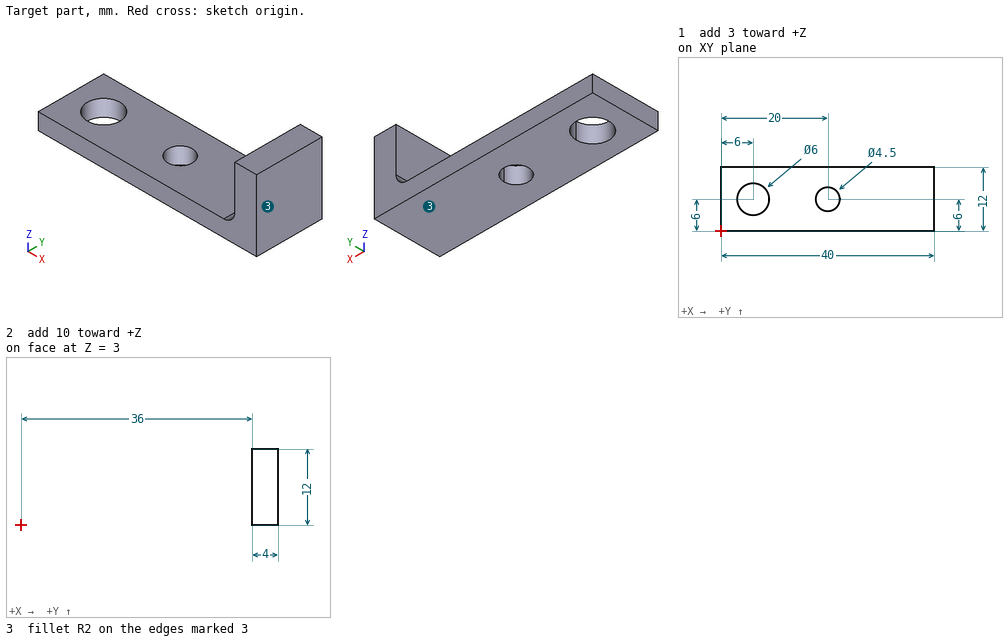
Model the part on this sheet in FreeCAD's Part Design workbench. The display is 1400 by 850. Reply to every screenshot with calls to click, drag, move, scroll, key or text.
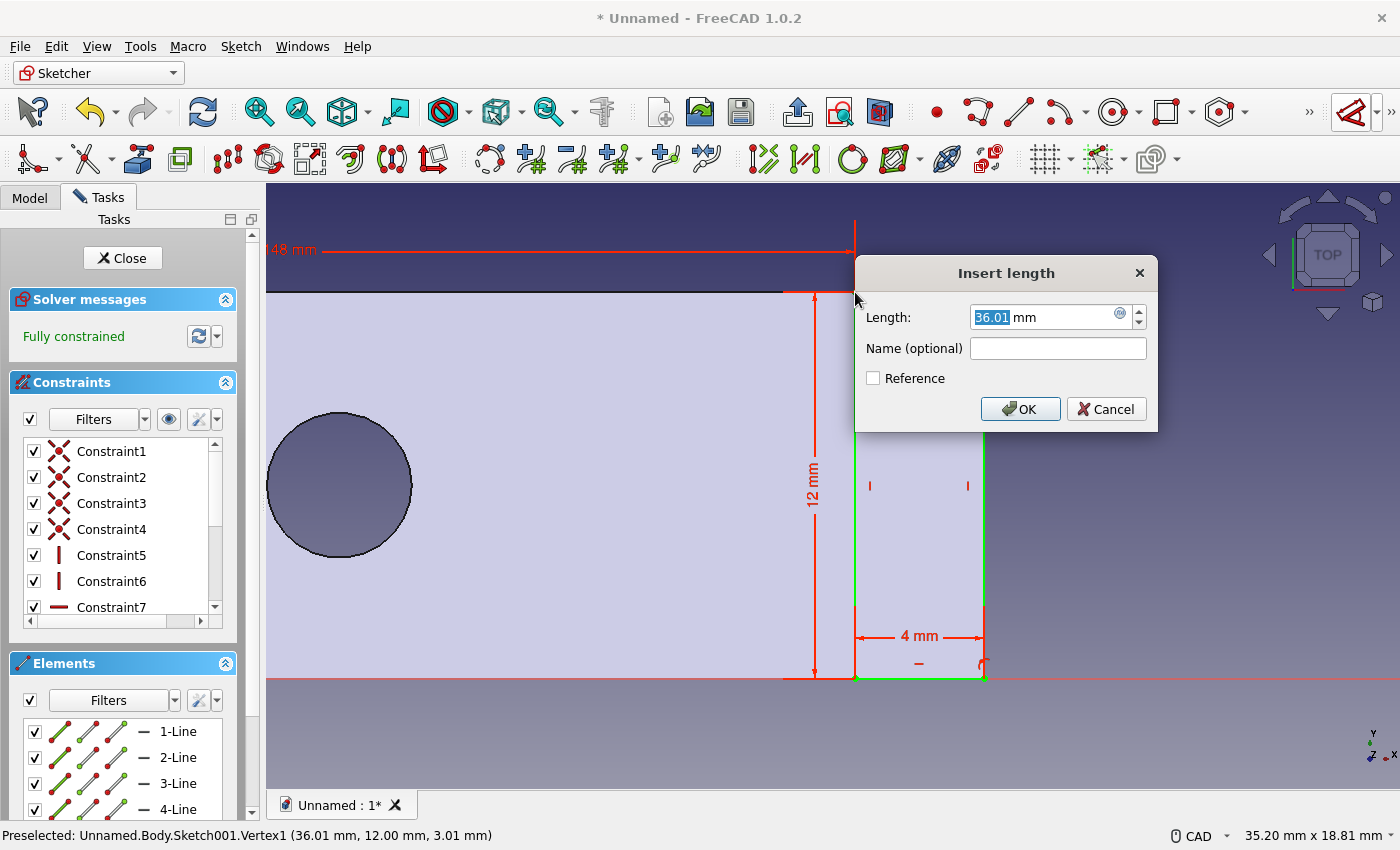
text(36)
key(Return)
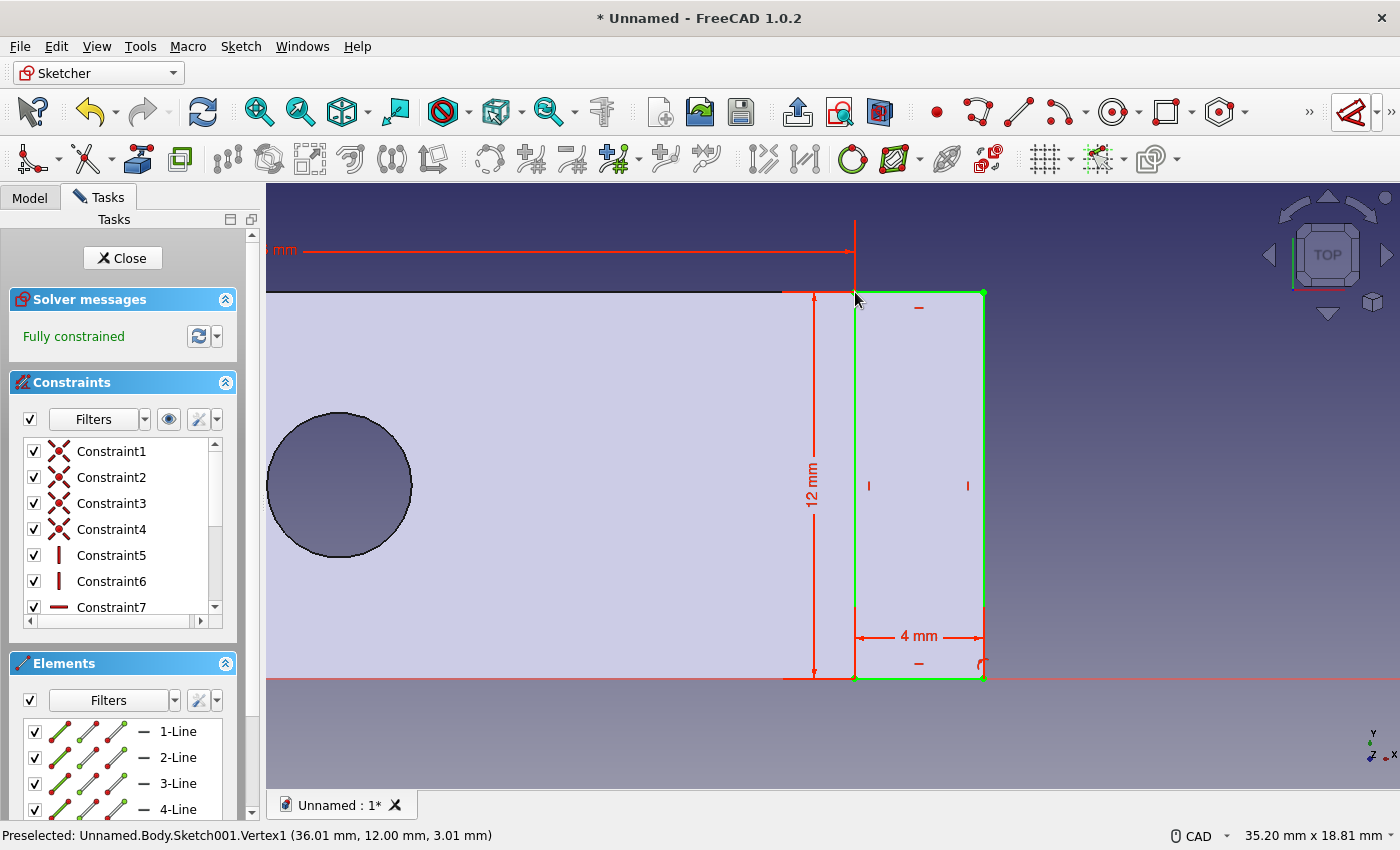
click(123, 258)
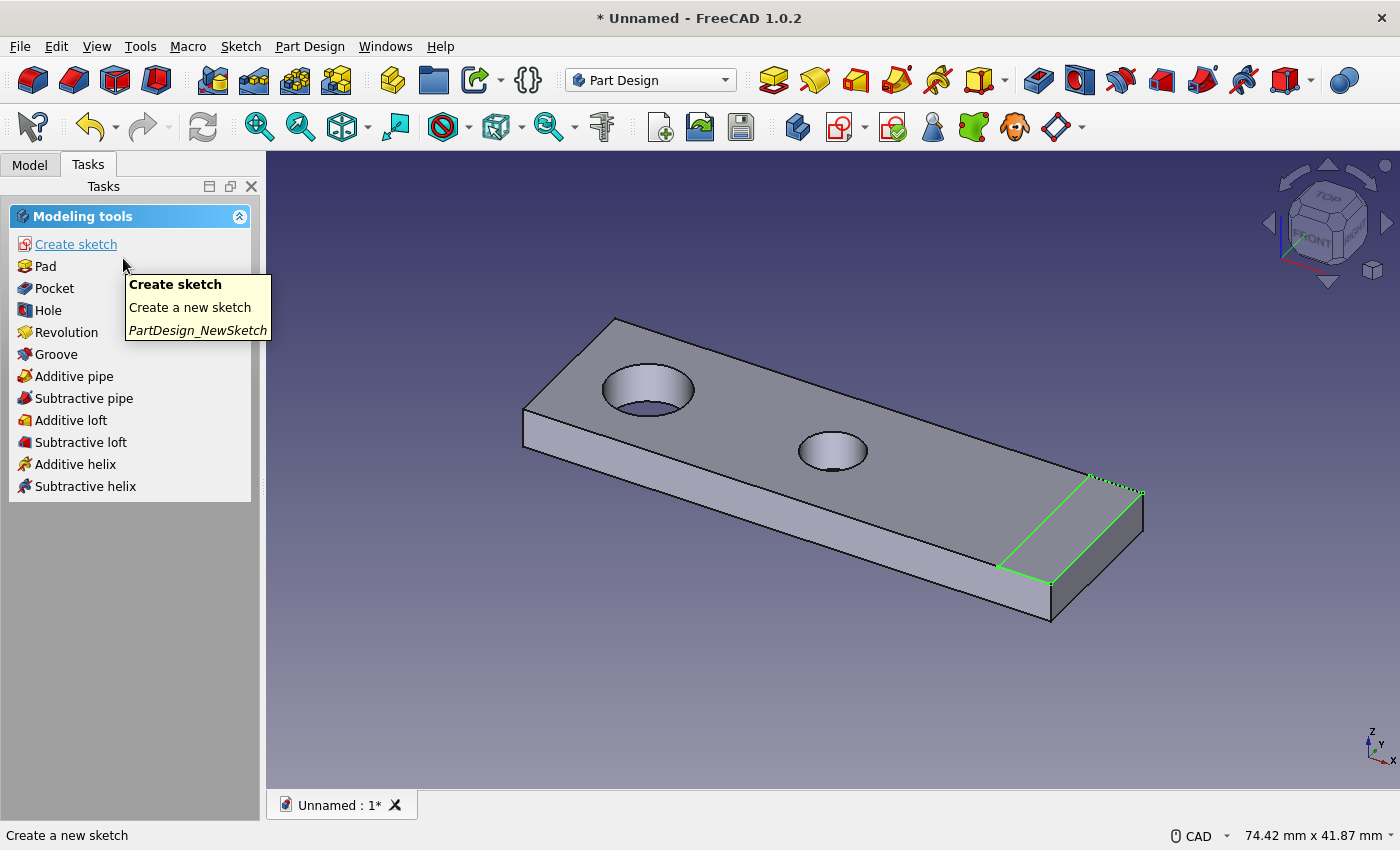
click(774, 80)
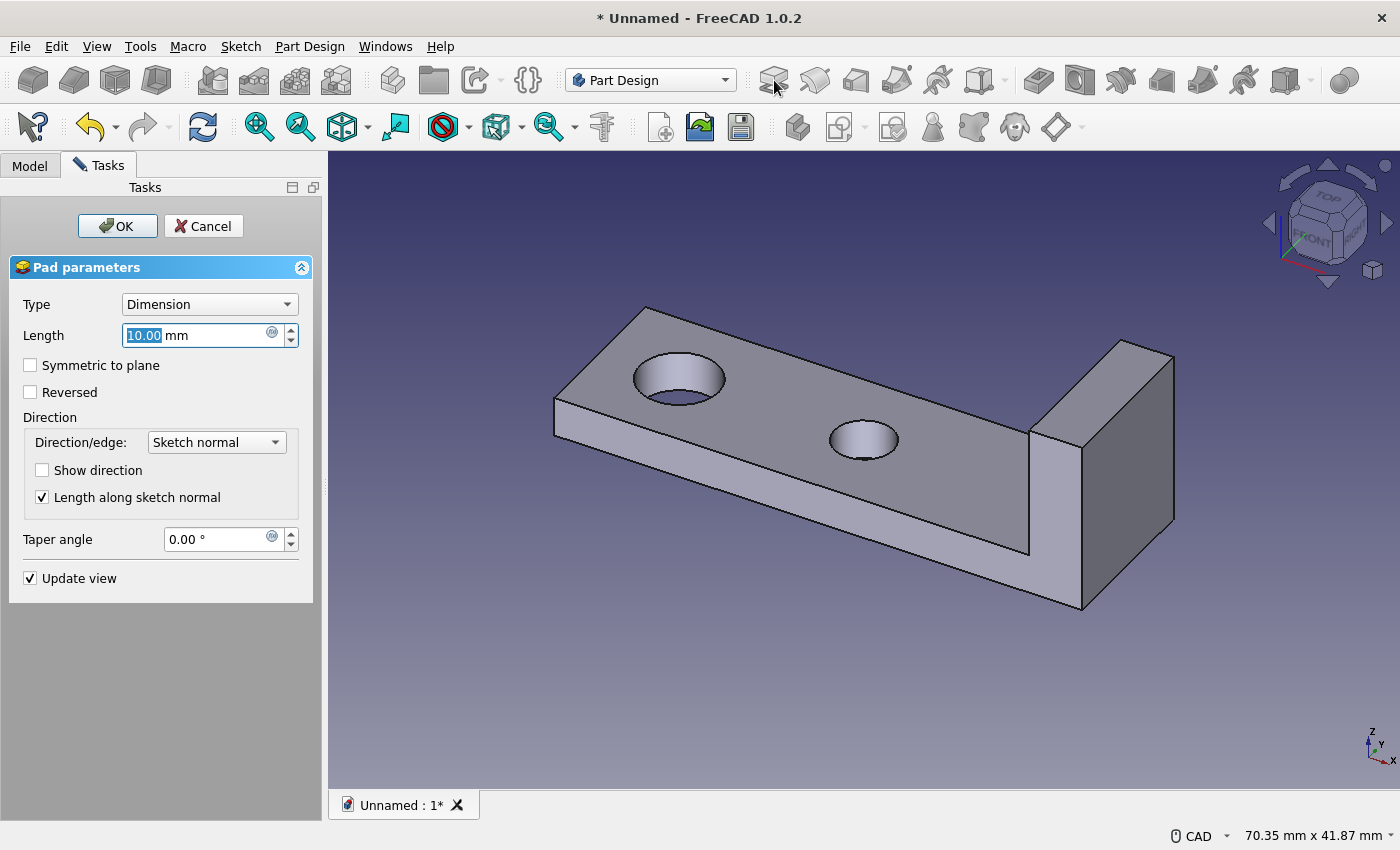
text(10)
key(Tab)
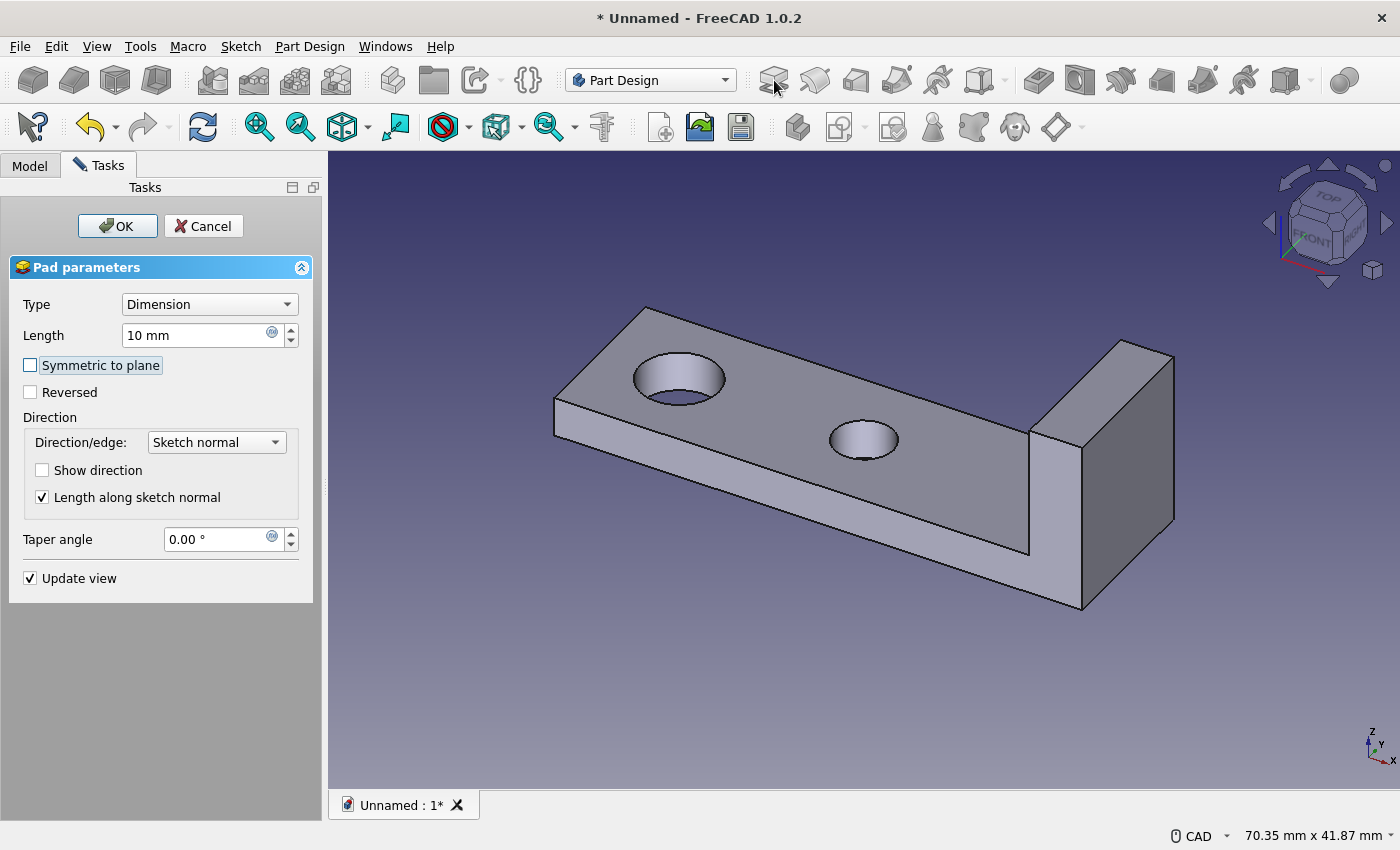
click(118, 226)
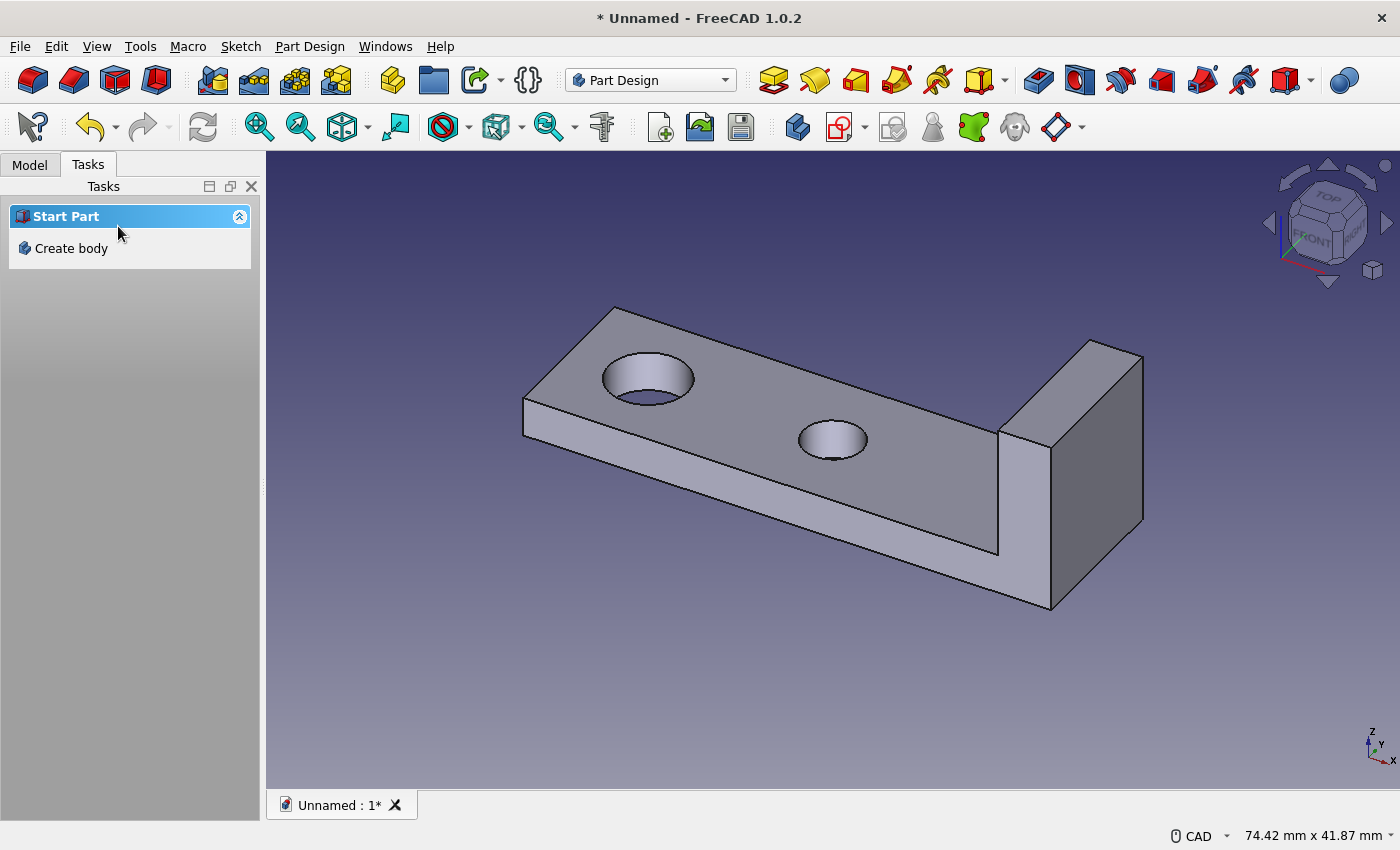
key(0)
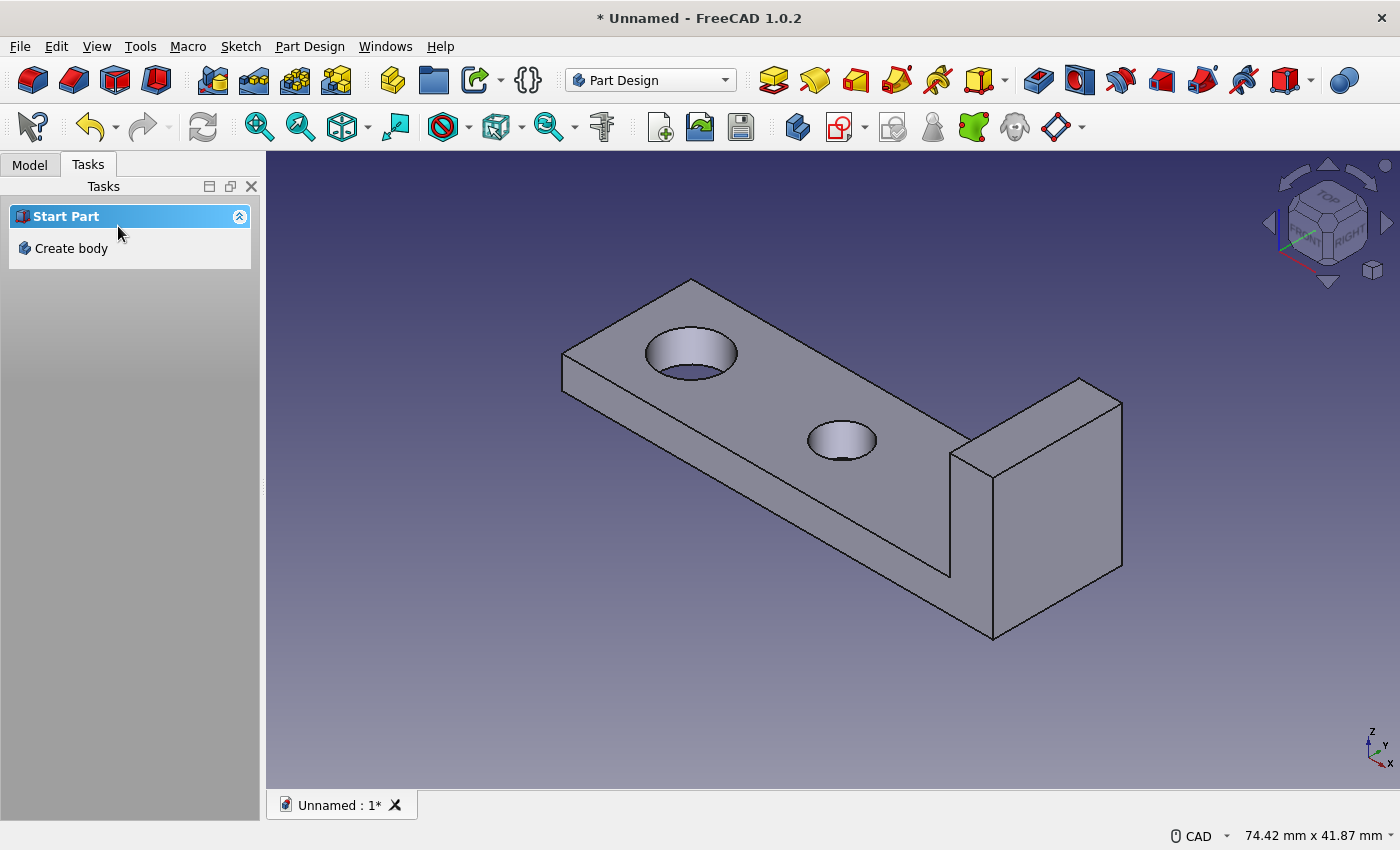
key(2)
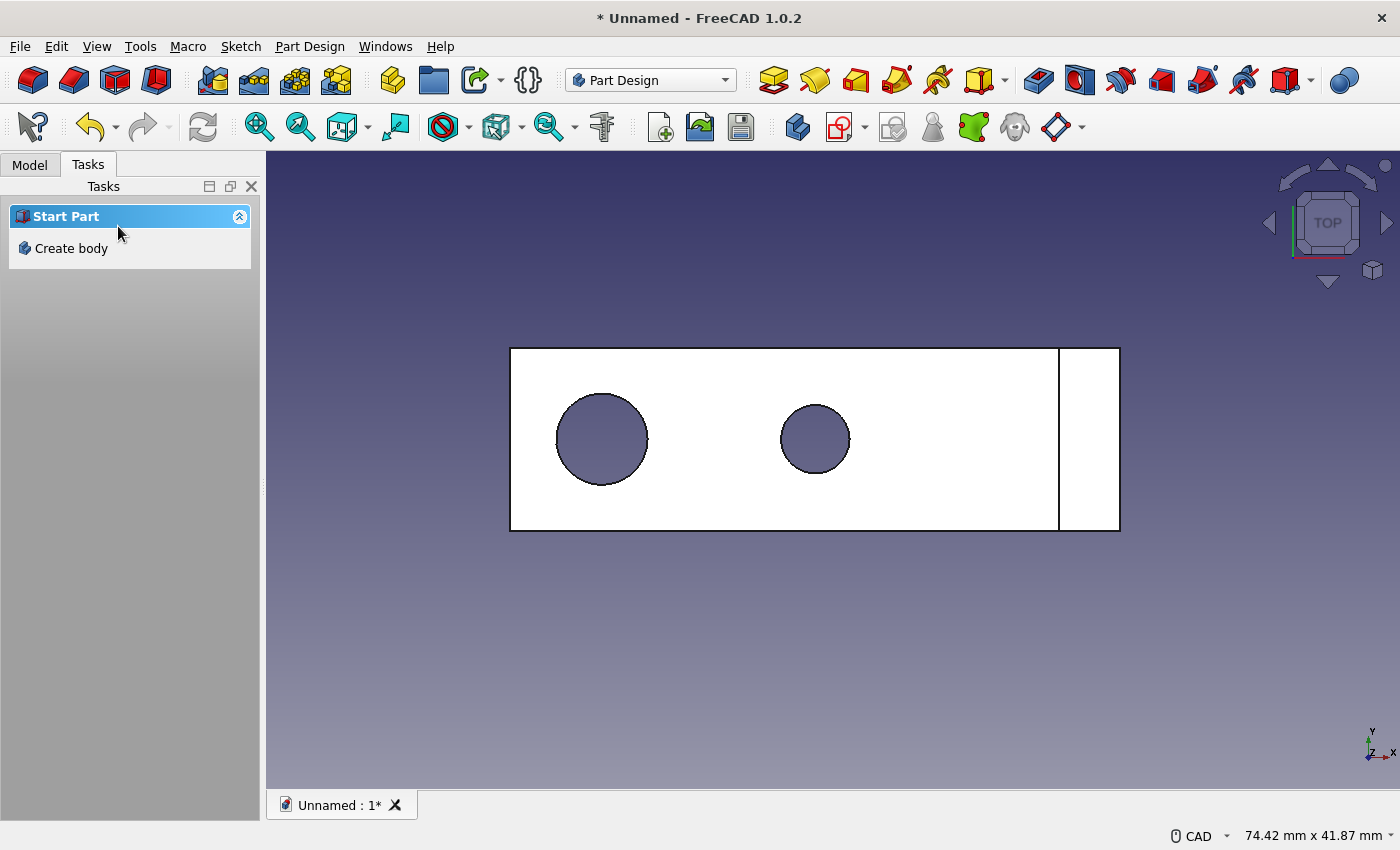
key(1)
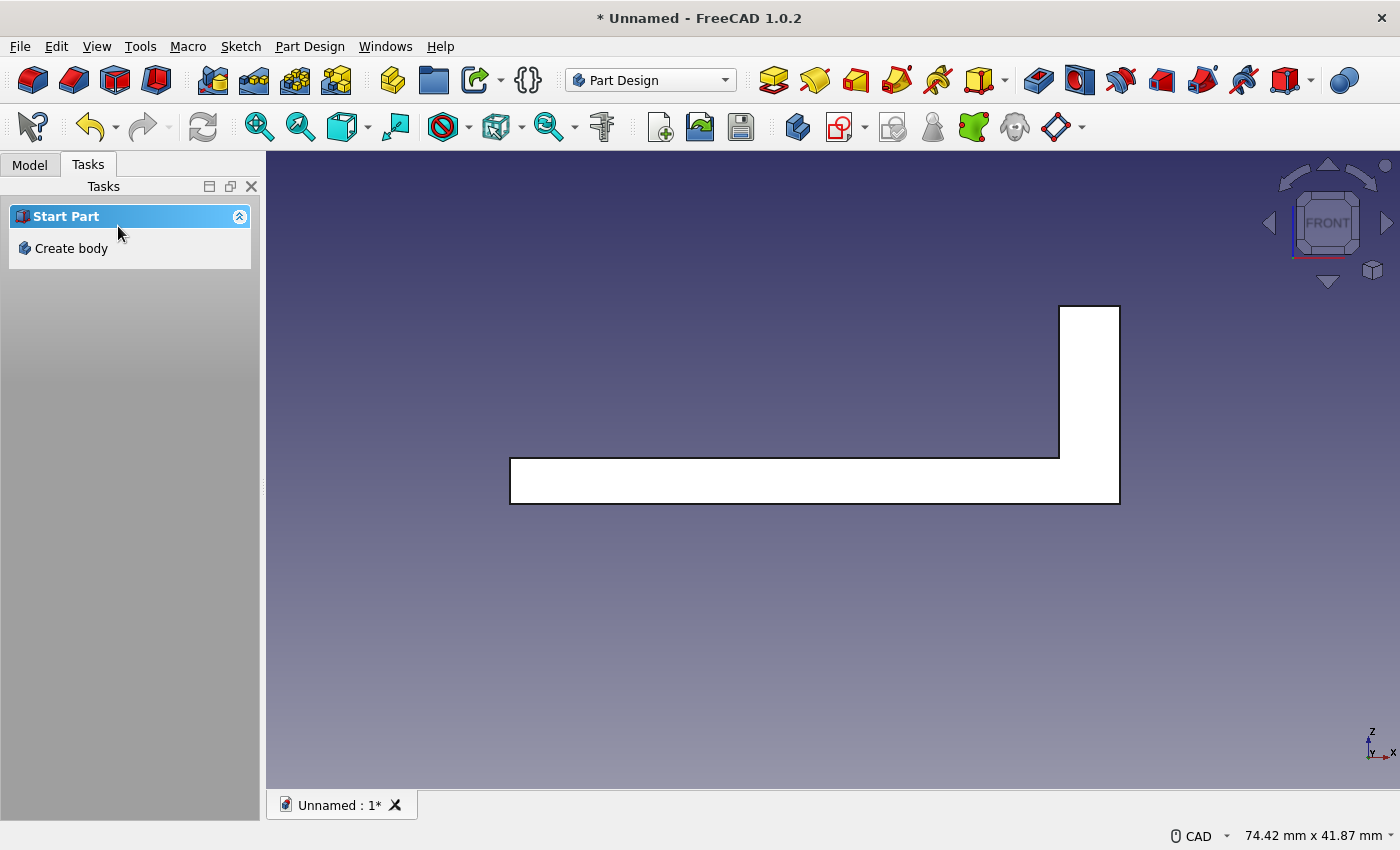
key(3)